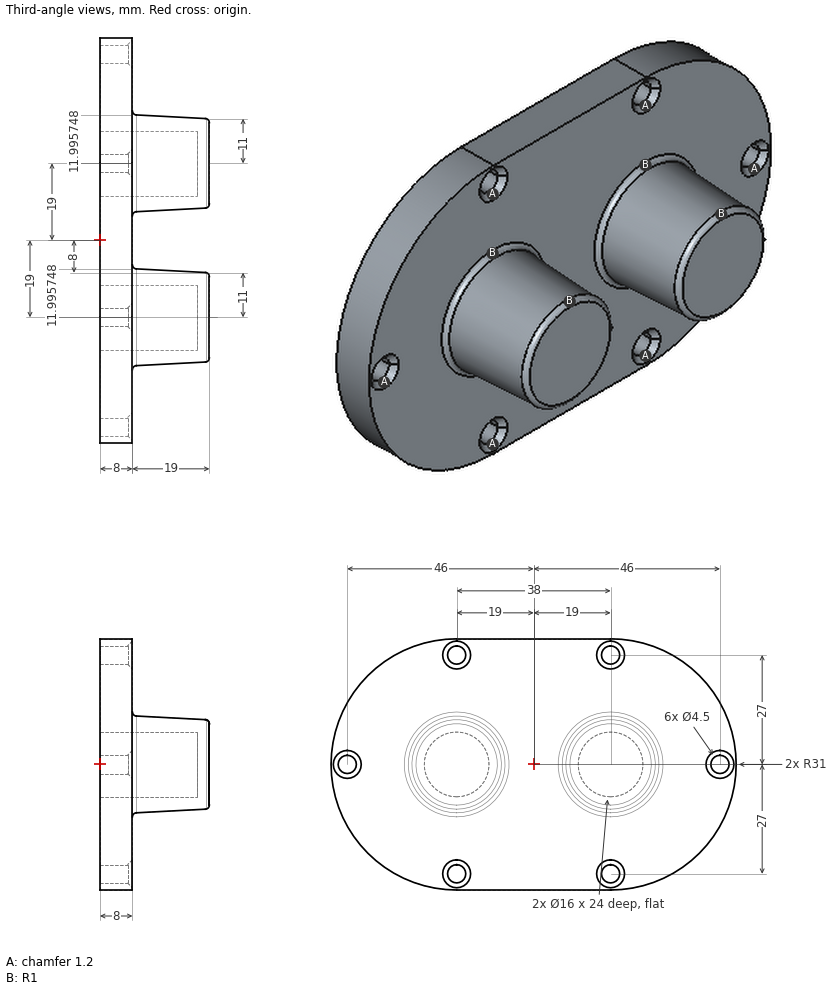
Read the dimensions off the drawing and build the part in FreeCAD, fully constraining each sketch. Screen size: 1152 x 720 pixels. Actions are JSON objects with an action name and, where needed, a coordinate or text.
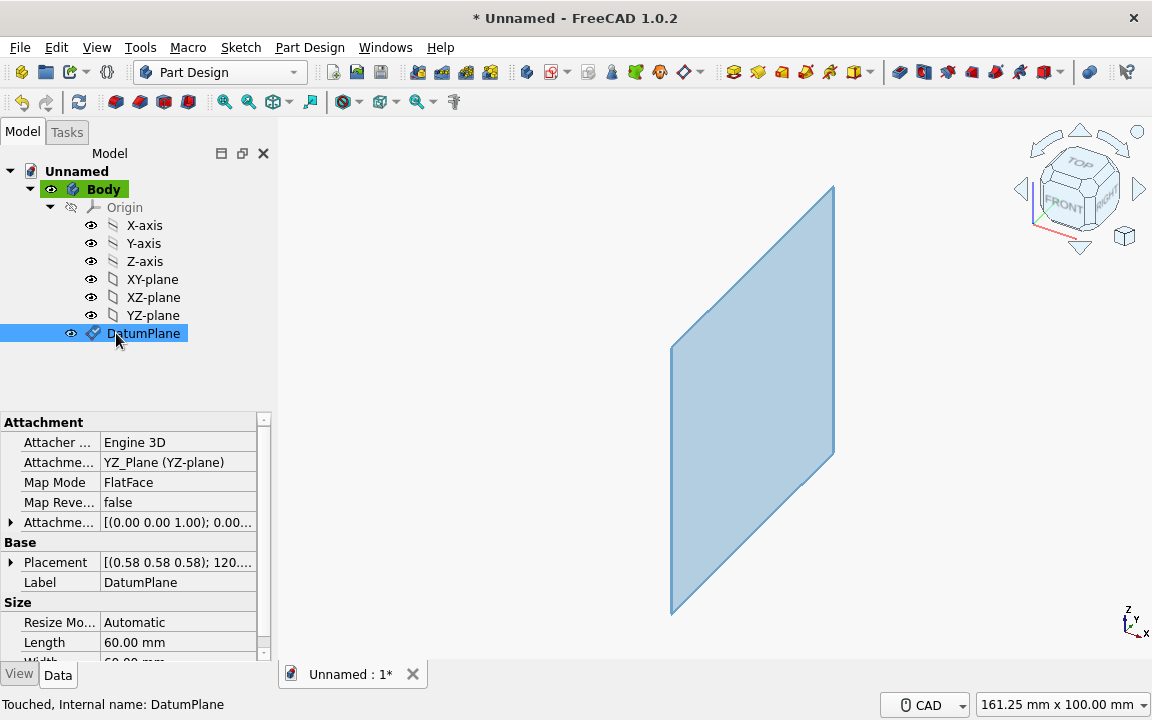
{"action": "left_click", "coordinate": [552, 72]}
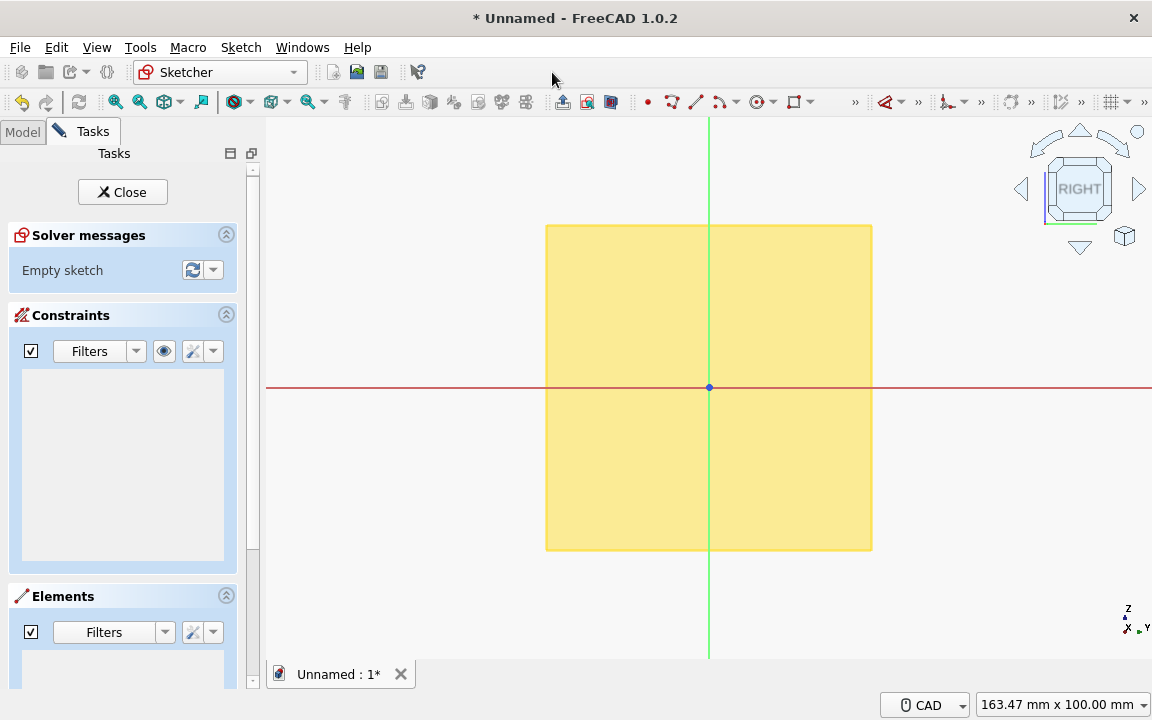
{"action": "scroll", "coordinate": [331, 388], "scroll_direction": "down", "scroll_amount": 1}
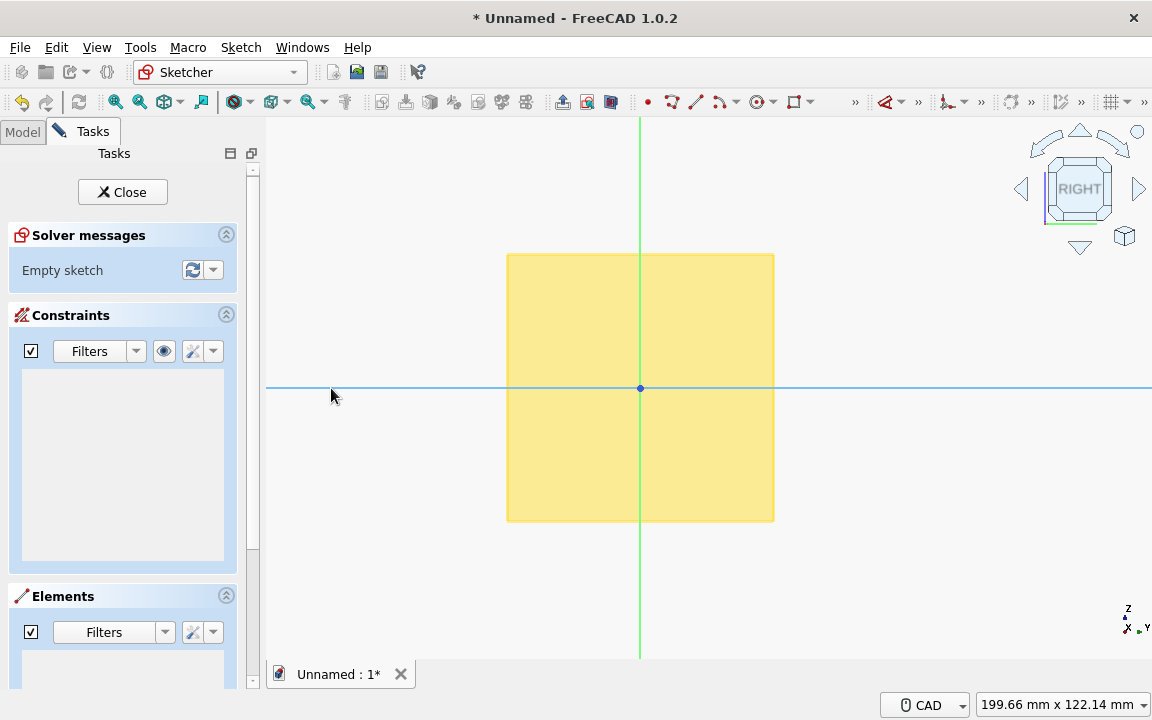
{"action": "key", "text": "g s"}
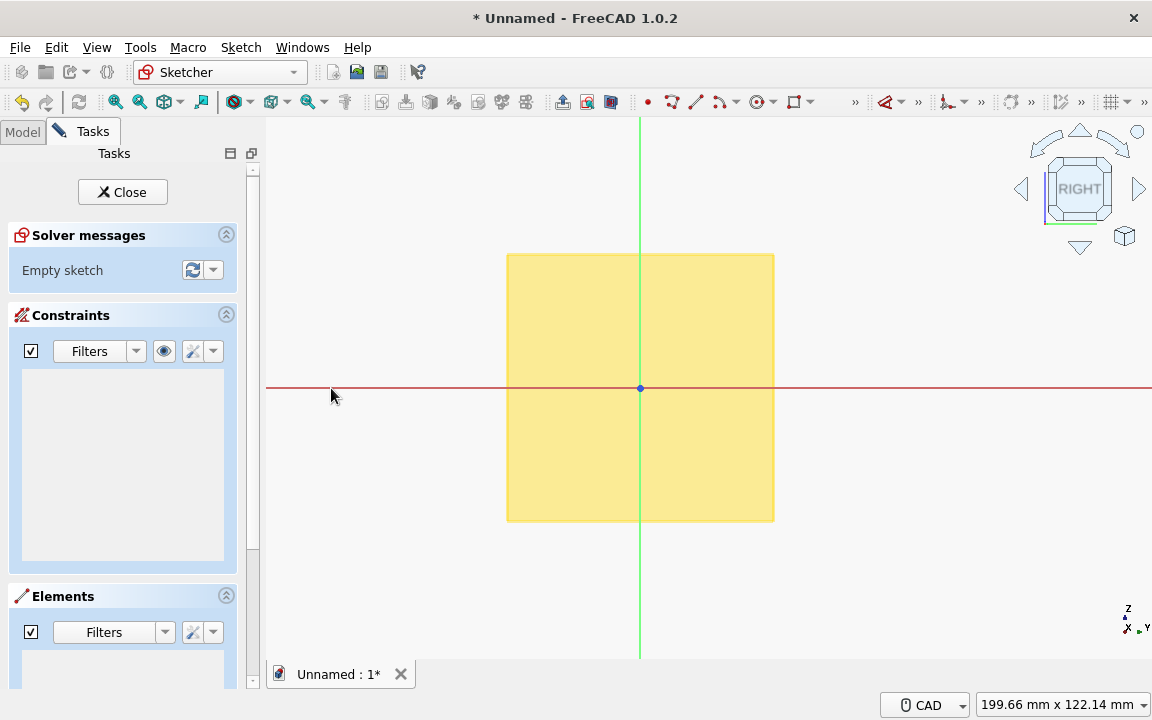
{"action": "left_click", "coordinate": [556, 388]}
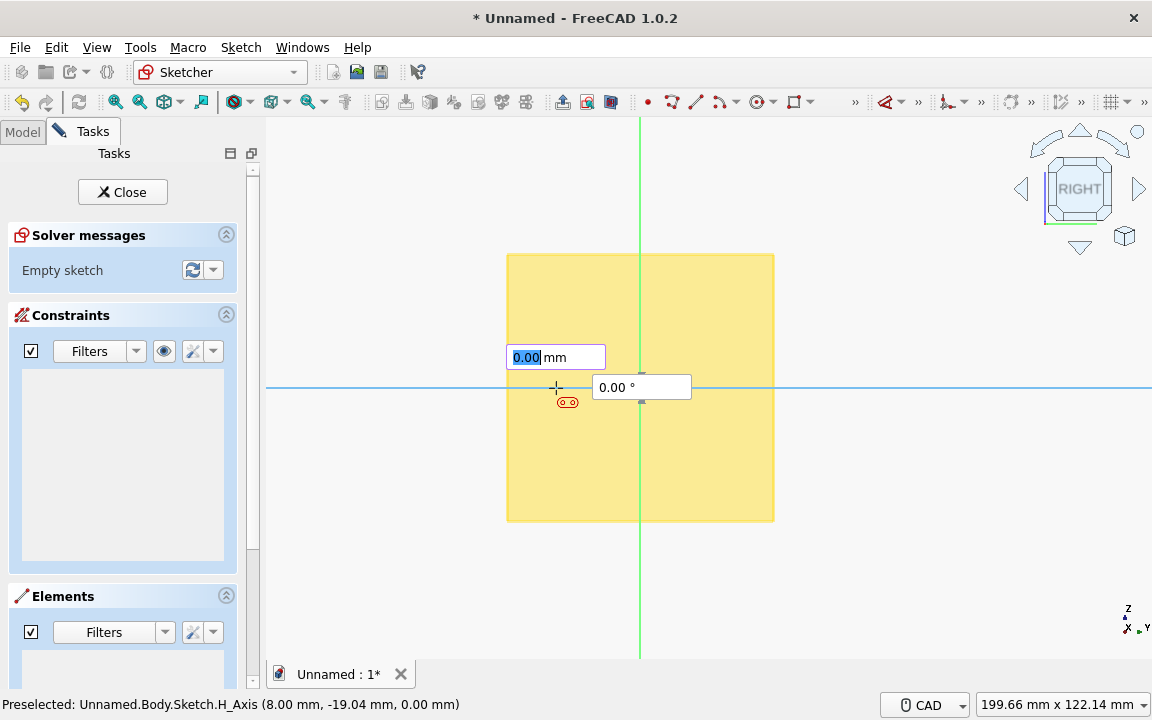
{"action": "left_click", "coordinate": [725, 379]}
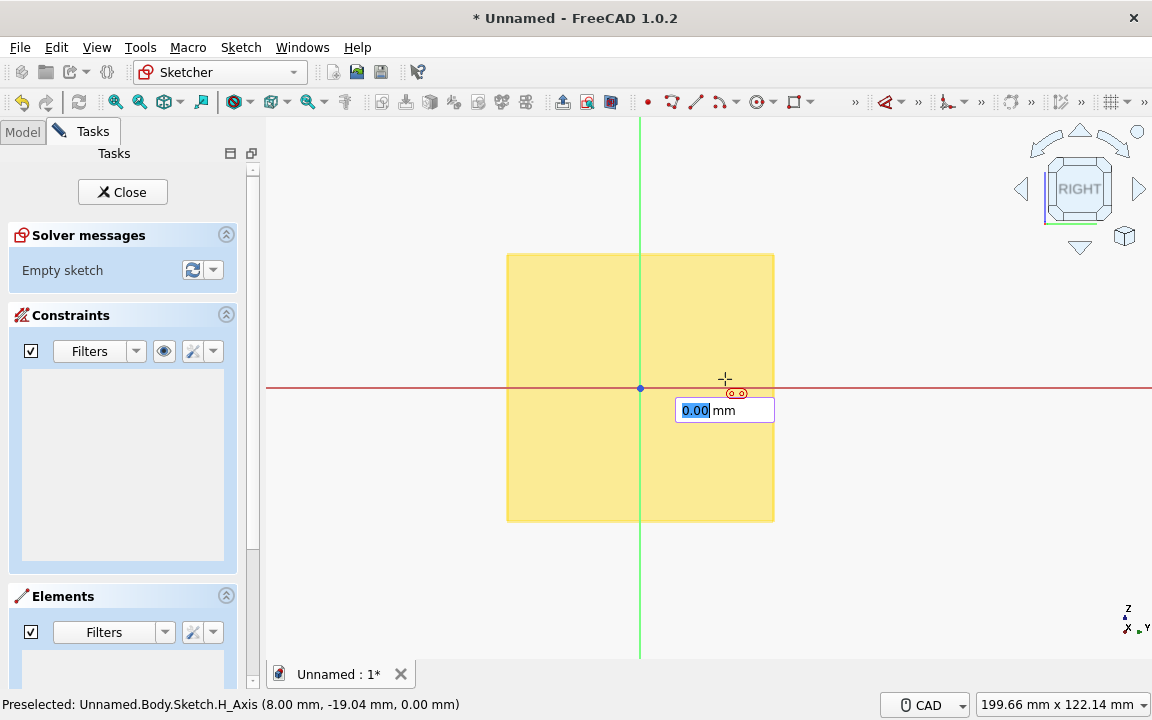
{"action": "left_click", "coordinate": [615, 526]}
{"action": "key", "text": "Escape"}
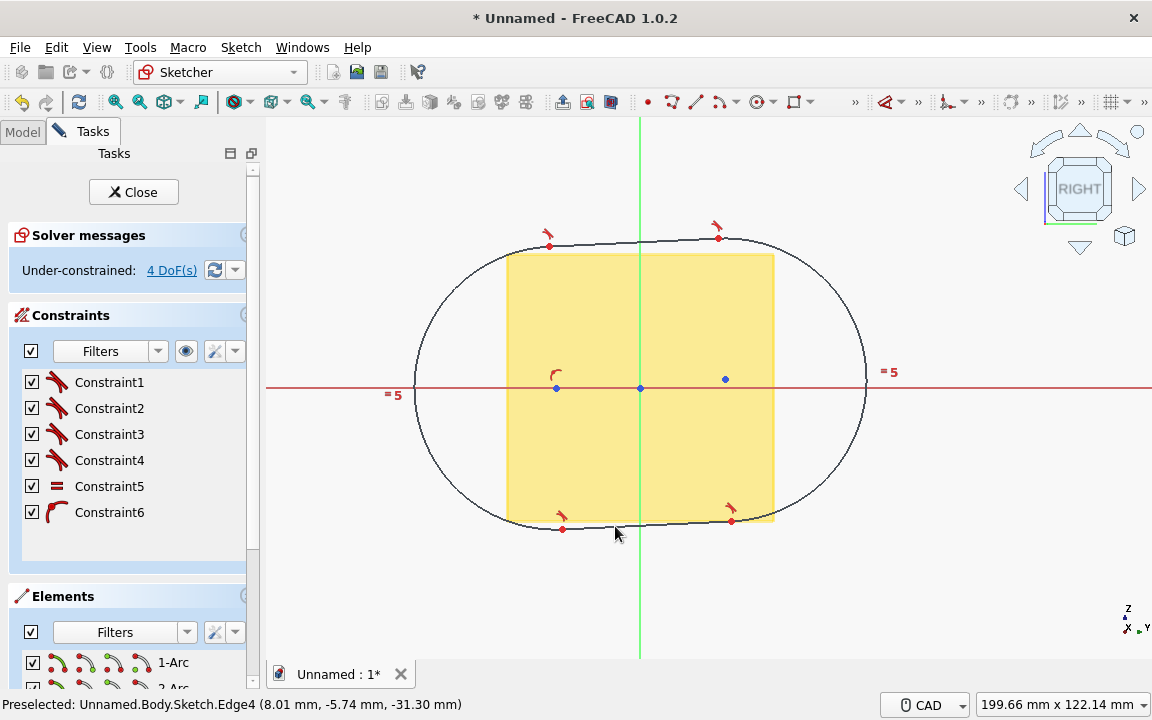
{"action": "left_click", "coordinate": [600, 244]}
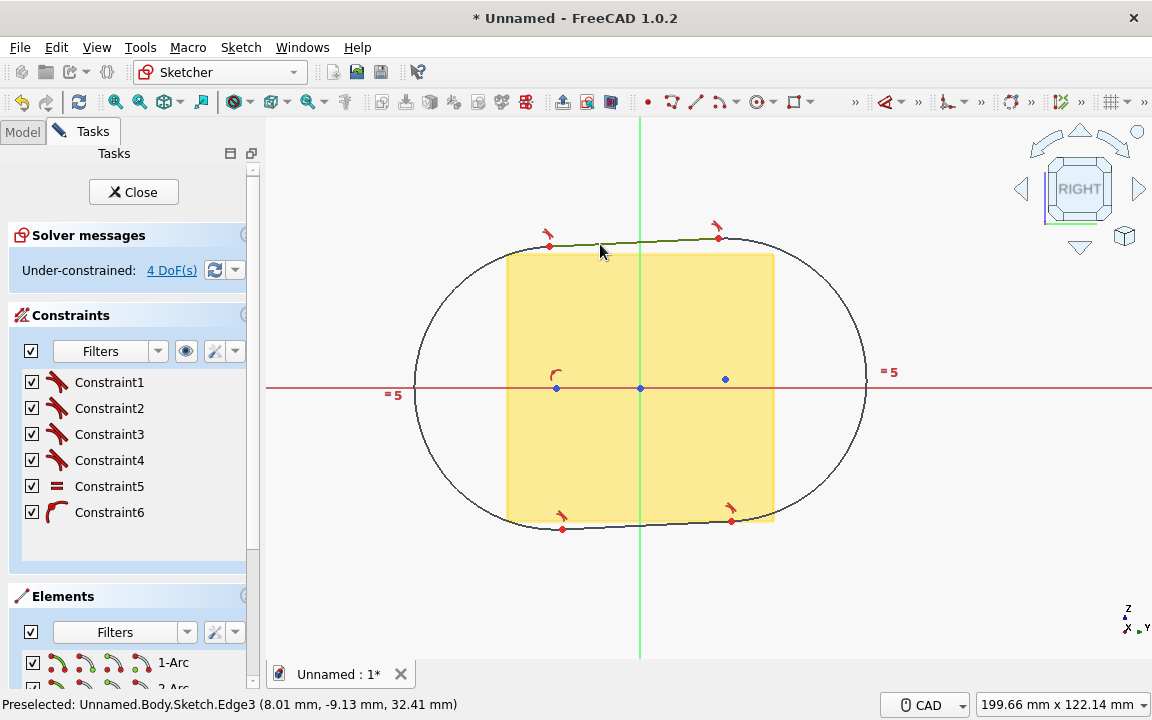
{"action": "key", "text": "h"}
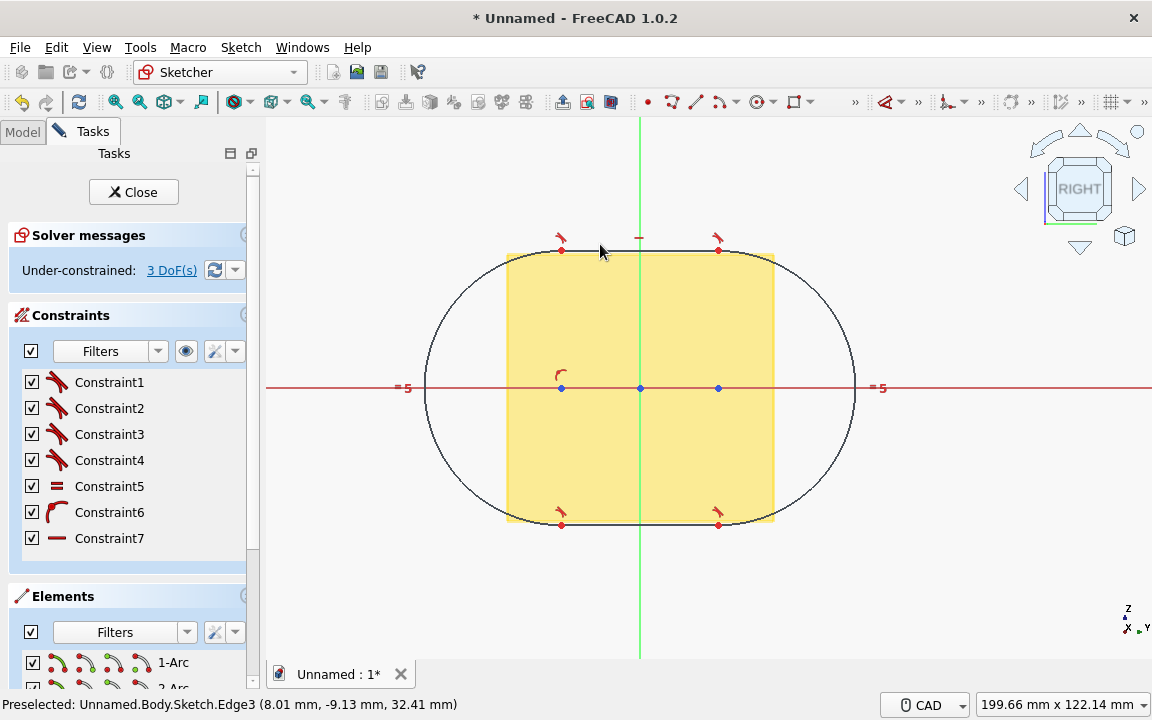
{"action": "left_click", "coordinate": [886, 102]}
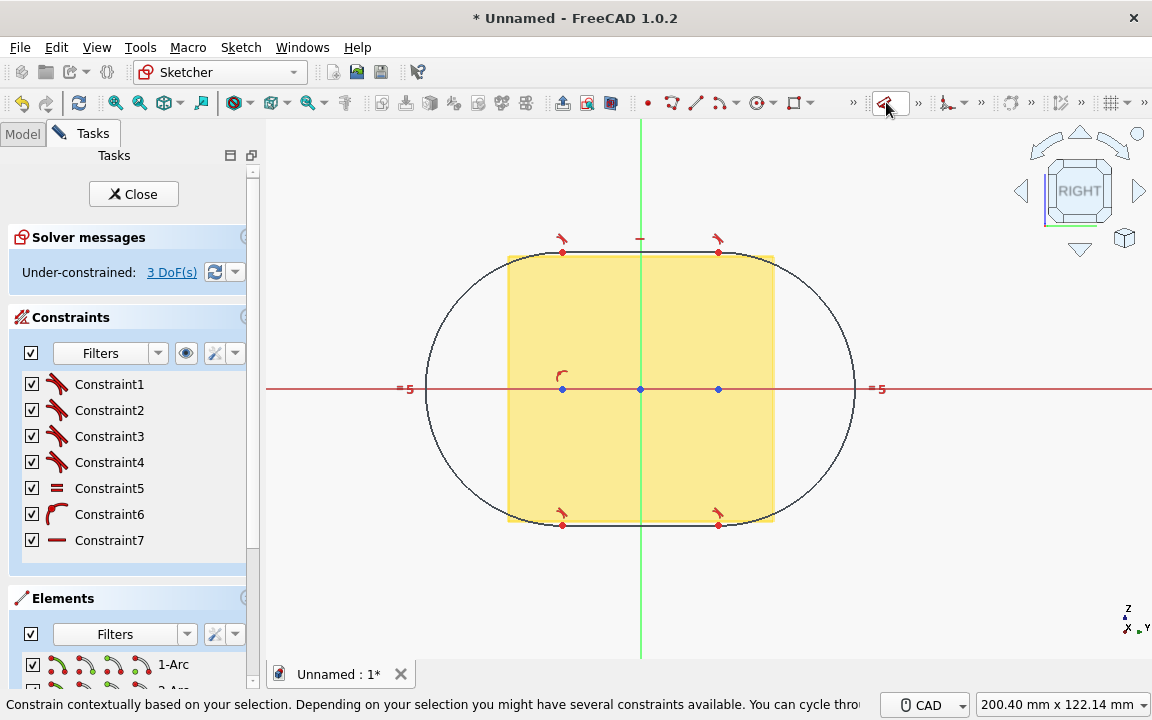
{"action": "left_click", "coordinate": [452, 309]}
{"action": "left_click", "coordinate": [426, 290]}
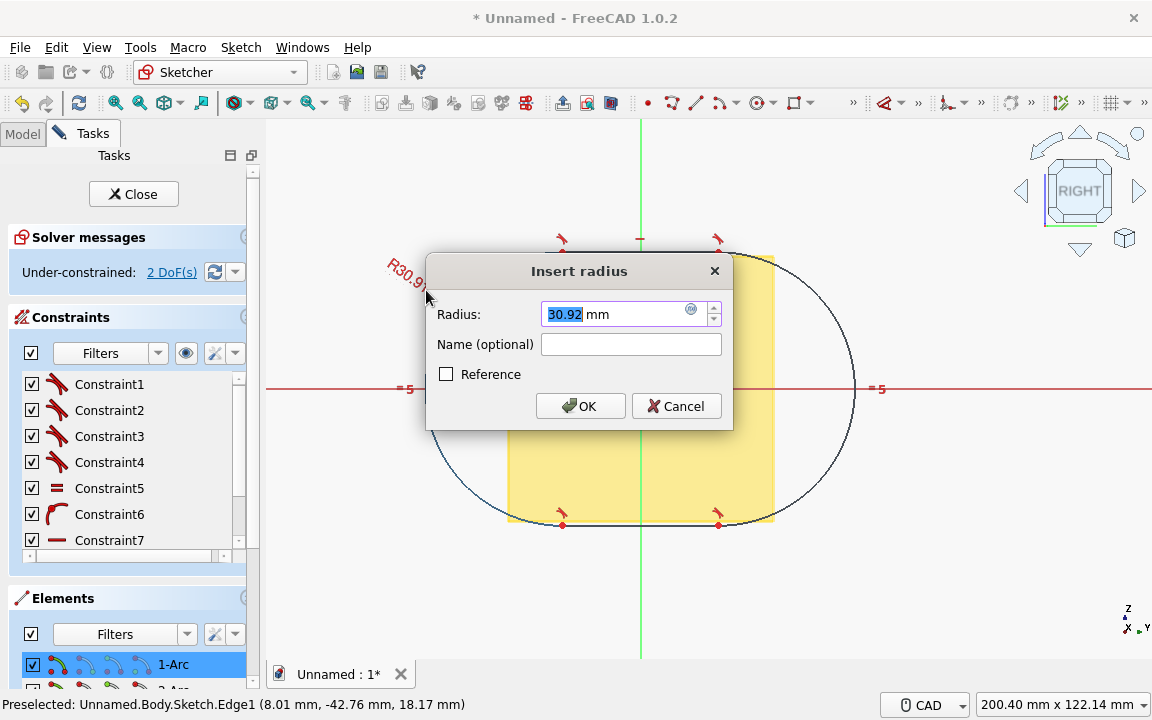
{"action": "type", "text": "31"}
{"action": "key", "text": "Return"}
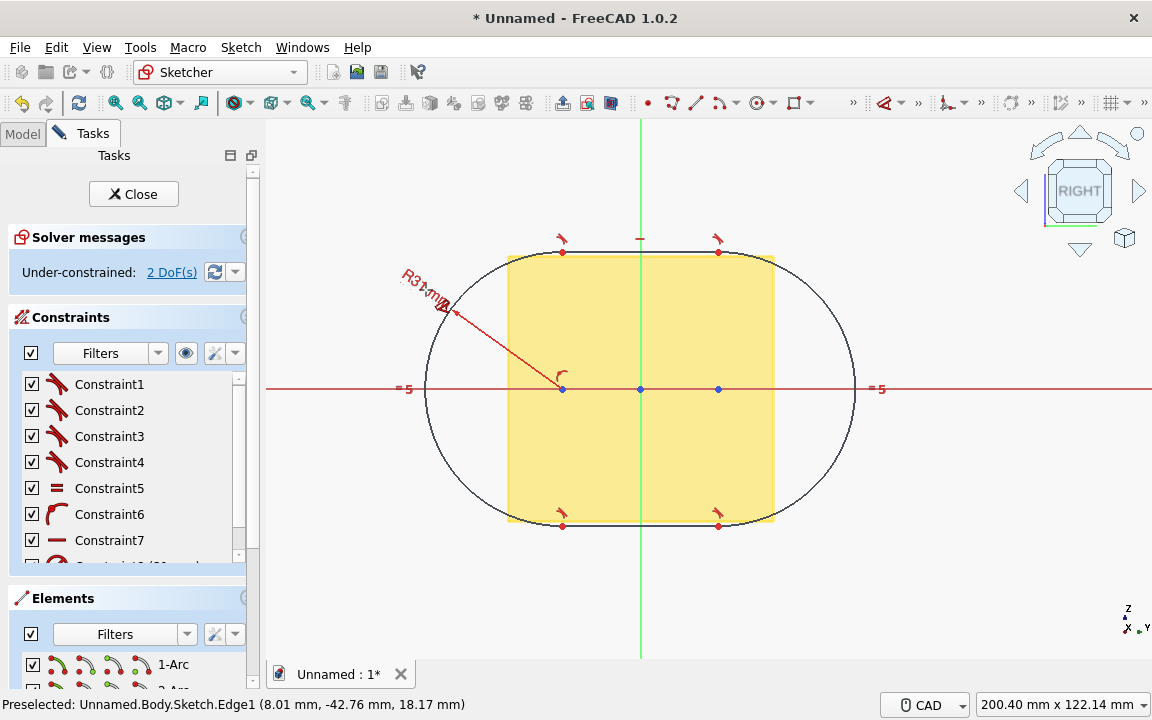
{"action": "left_click", "coordinate": [609, 252]}
{"action": "left_click", "coordinate": [604, 218]}